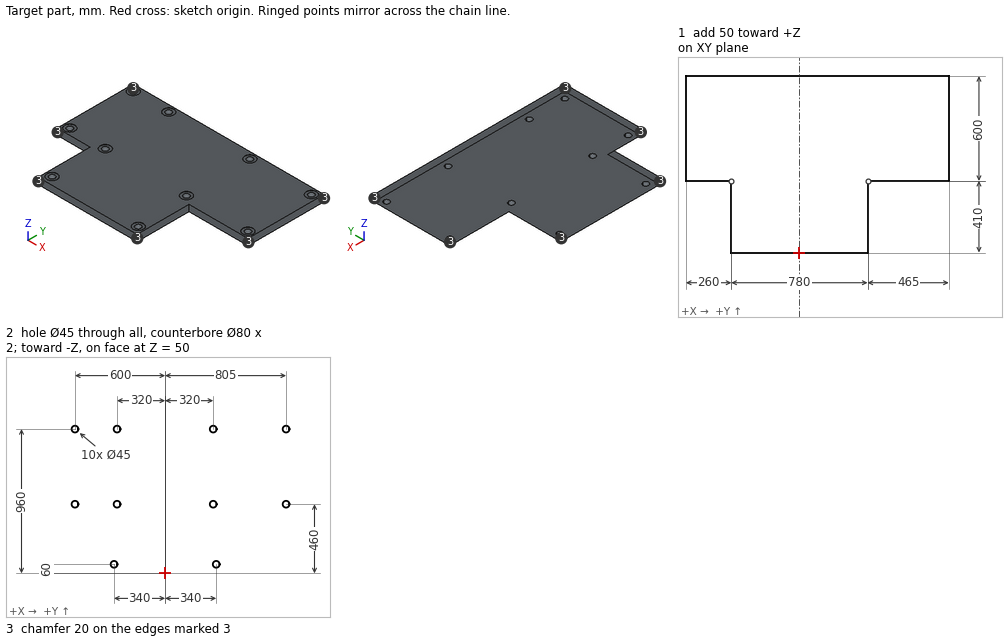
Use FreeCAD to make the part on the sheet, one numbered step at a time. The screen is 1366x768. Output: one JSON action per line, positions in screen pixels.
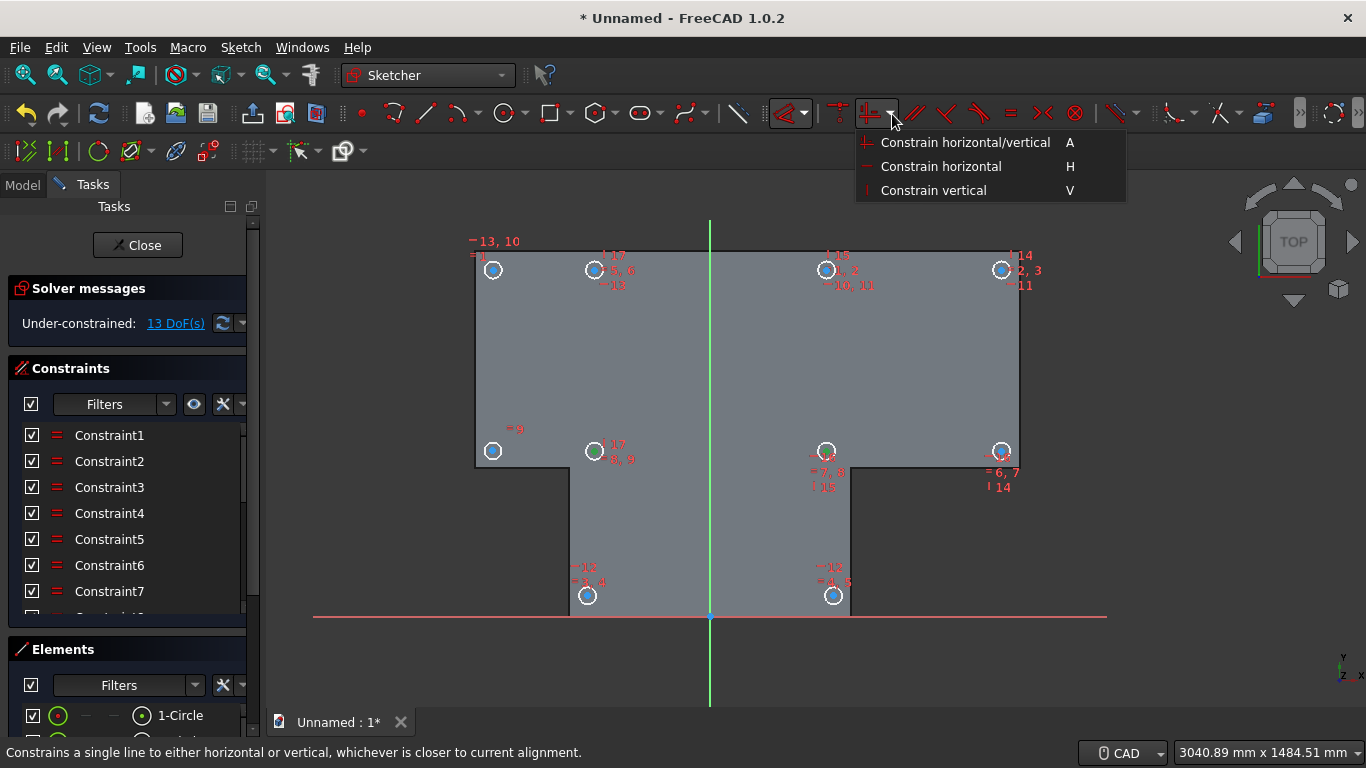
{"action": "left_click", "coordinate": [991, 166]}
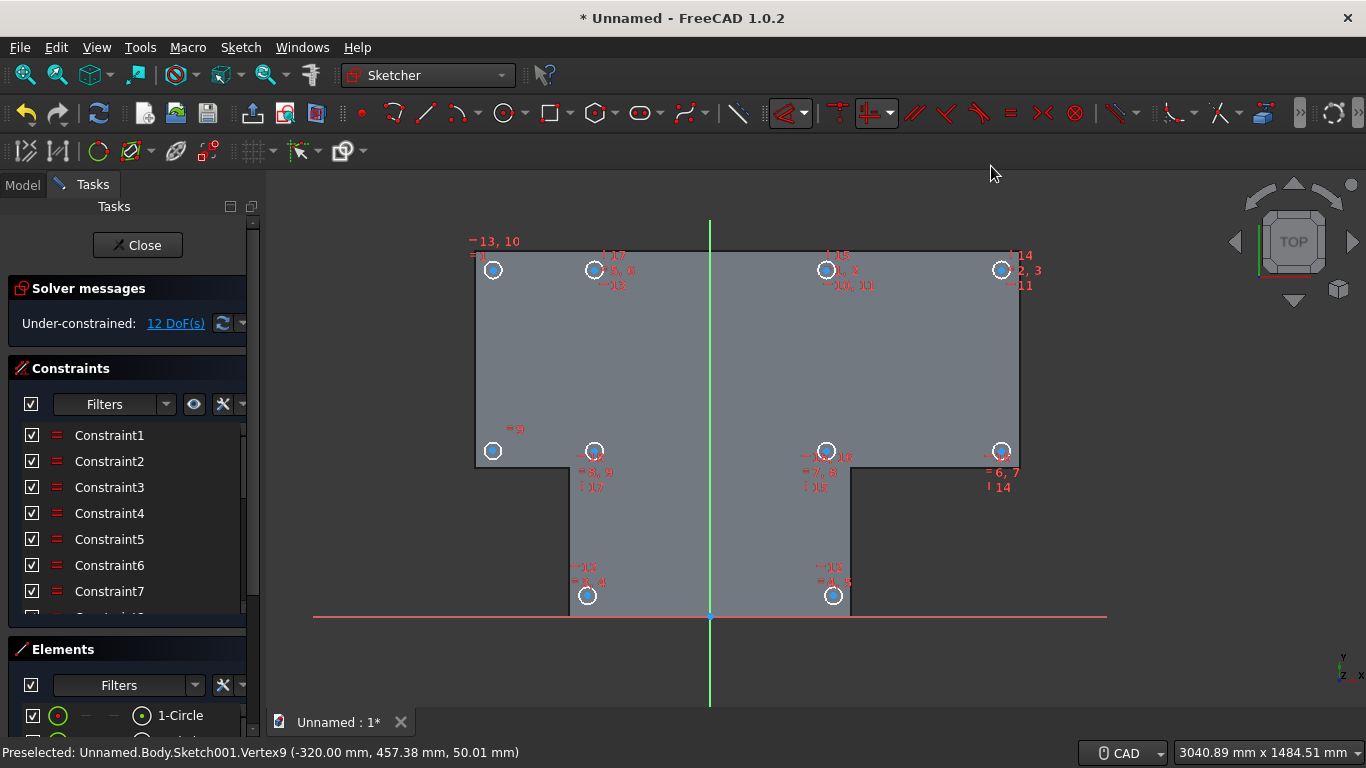
{"action": "left_click", "coordinate": [493, 270]}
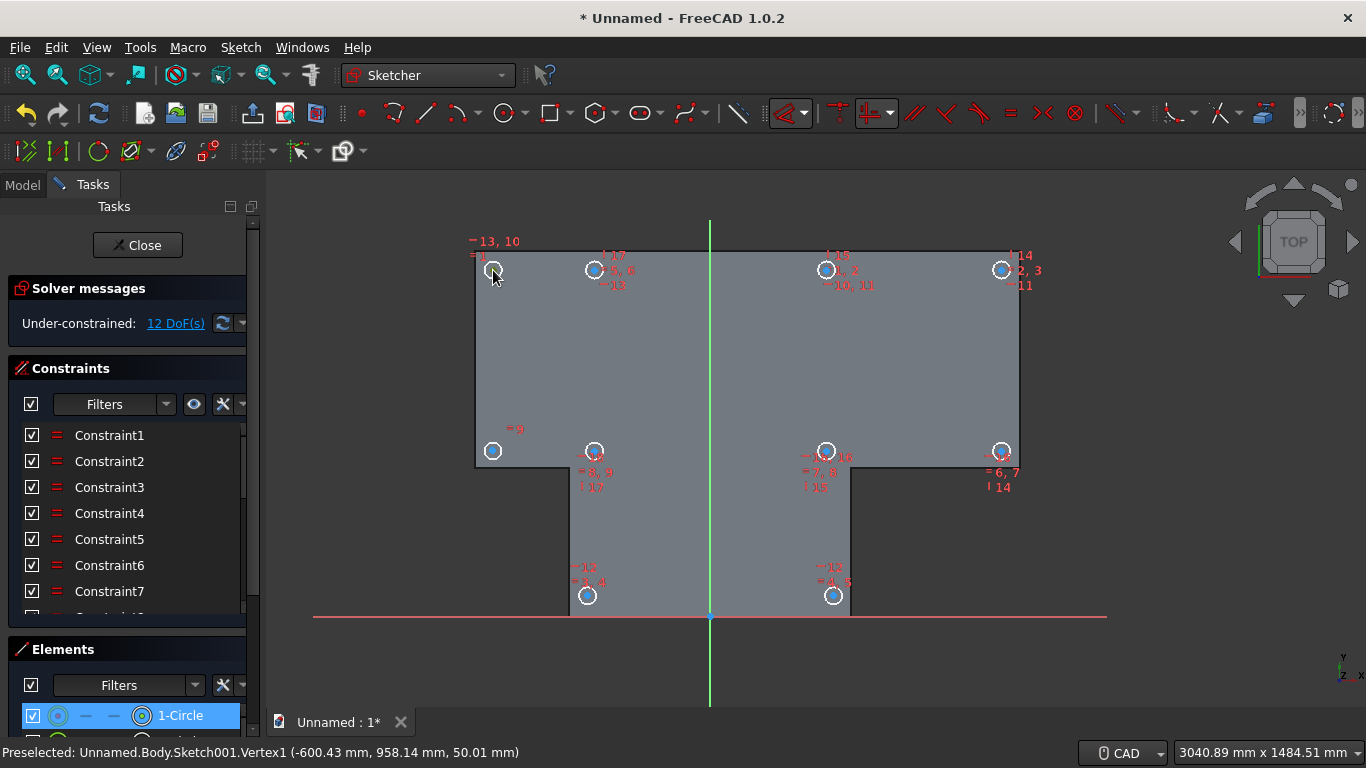
{"action": "left_click", "coordinate": [493, 451]}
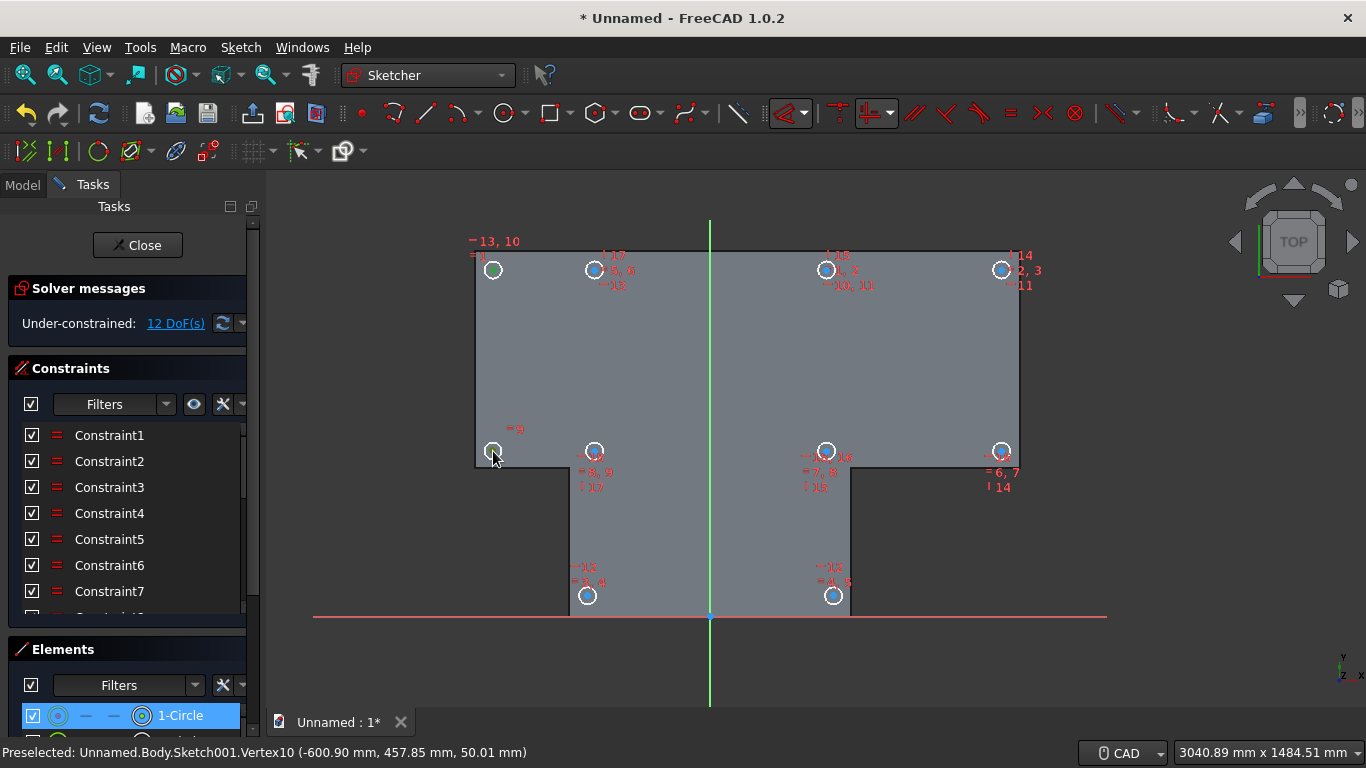
{"action": "left_click", "coordinate": [892, 114]}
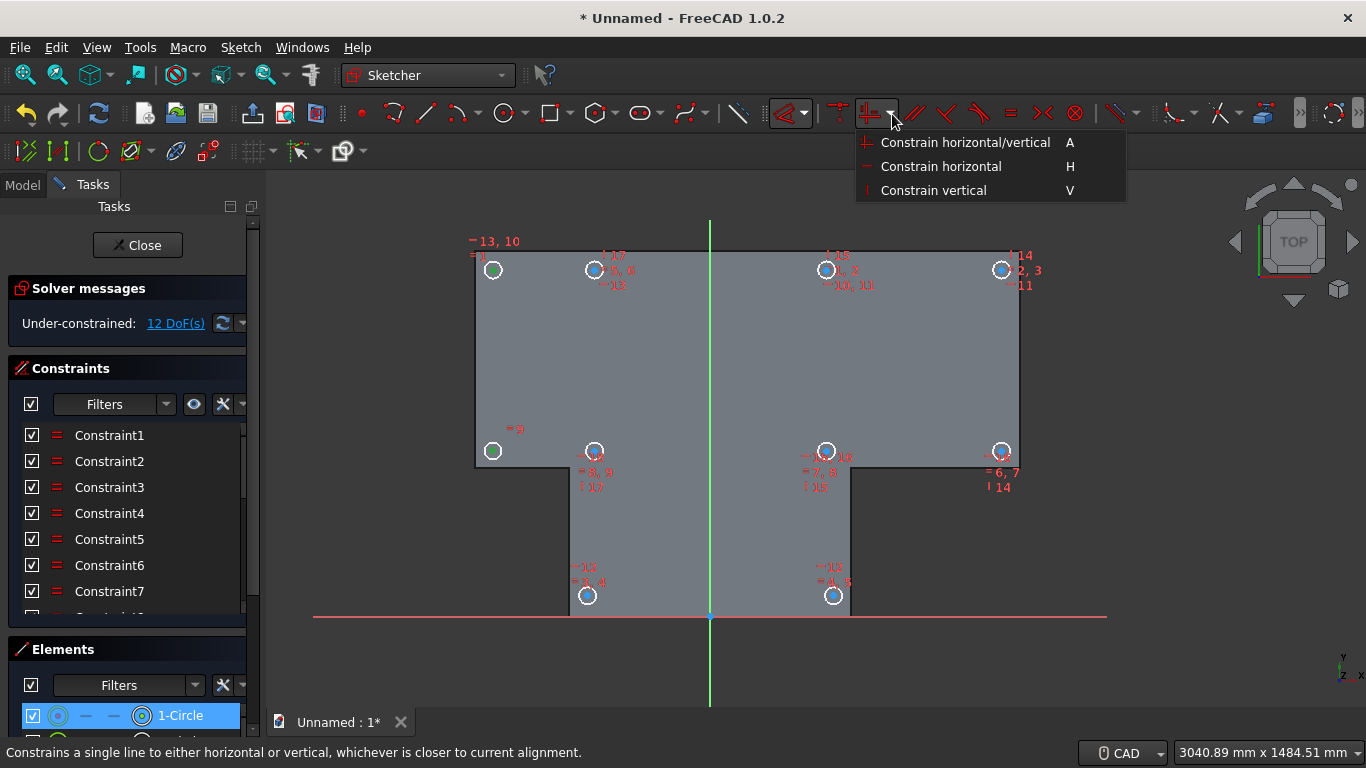
{"action": "left_click", "coordinate": [991, 190]}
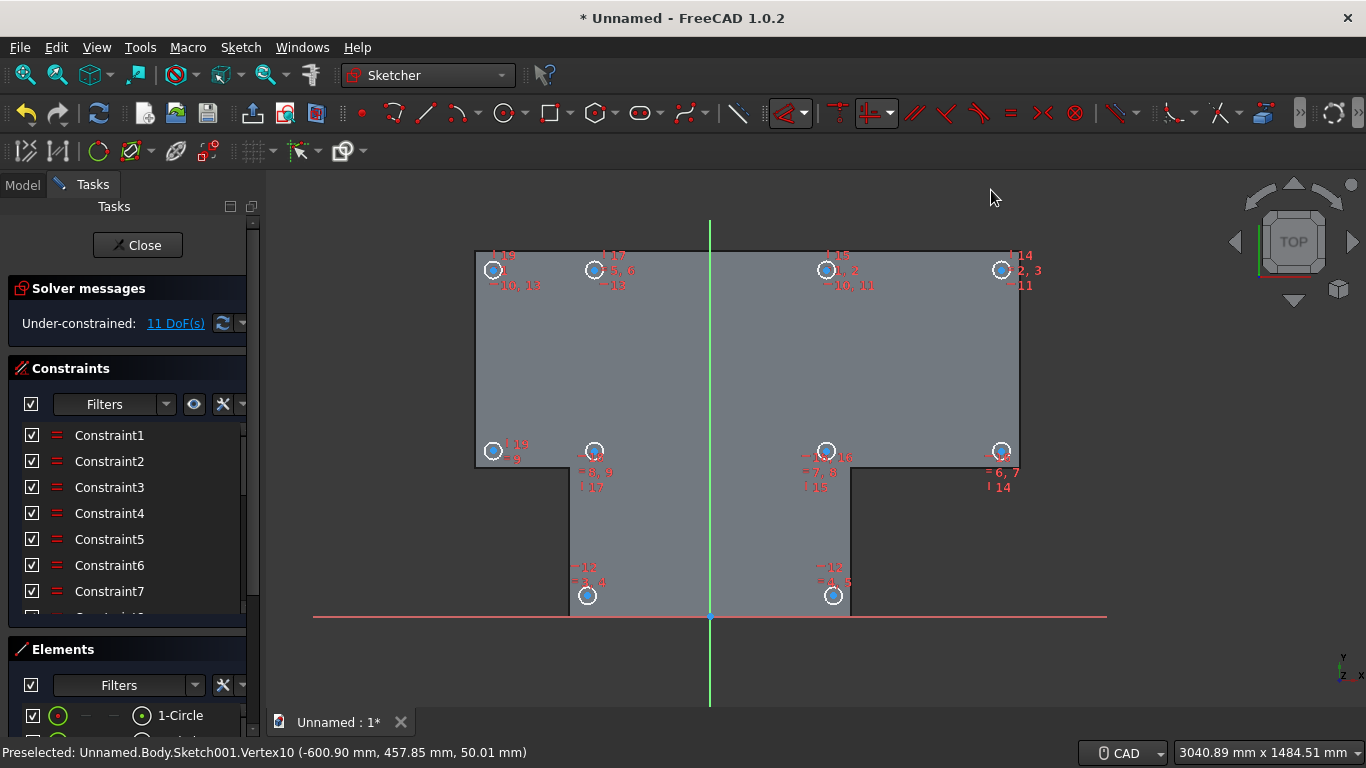
{"action": "left_click", "coordinate": [593, 449]}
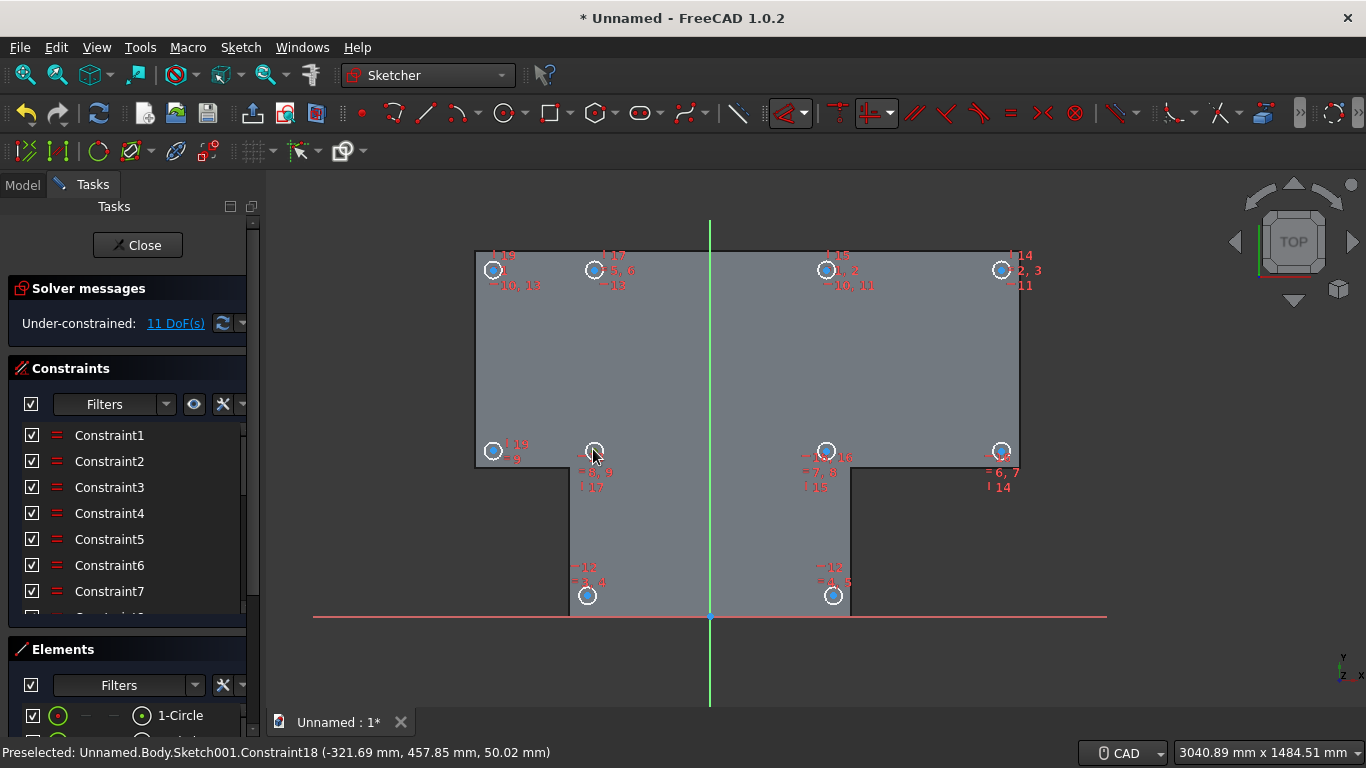
{"action": "left_click", "coordinate": [493, 451]}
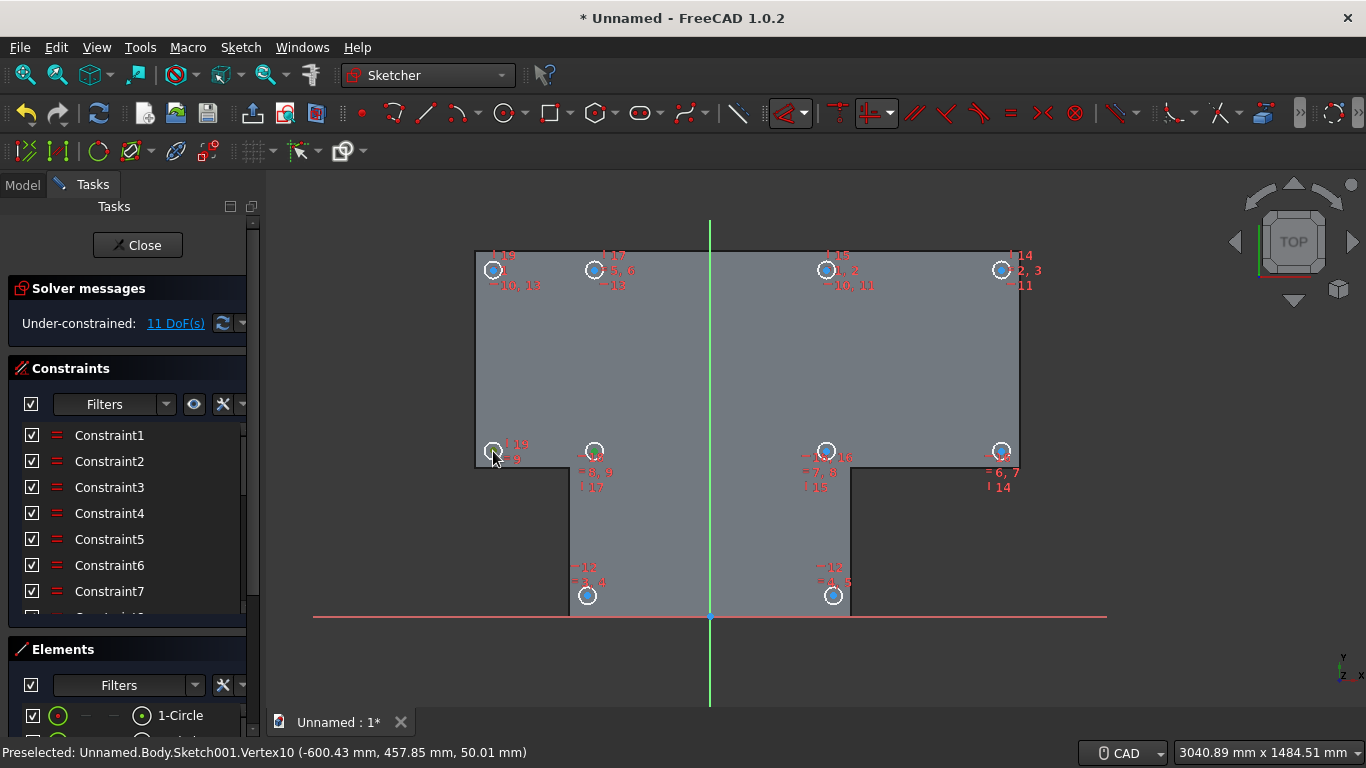
{"action": "key", "text": "h"}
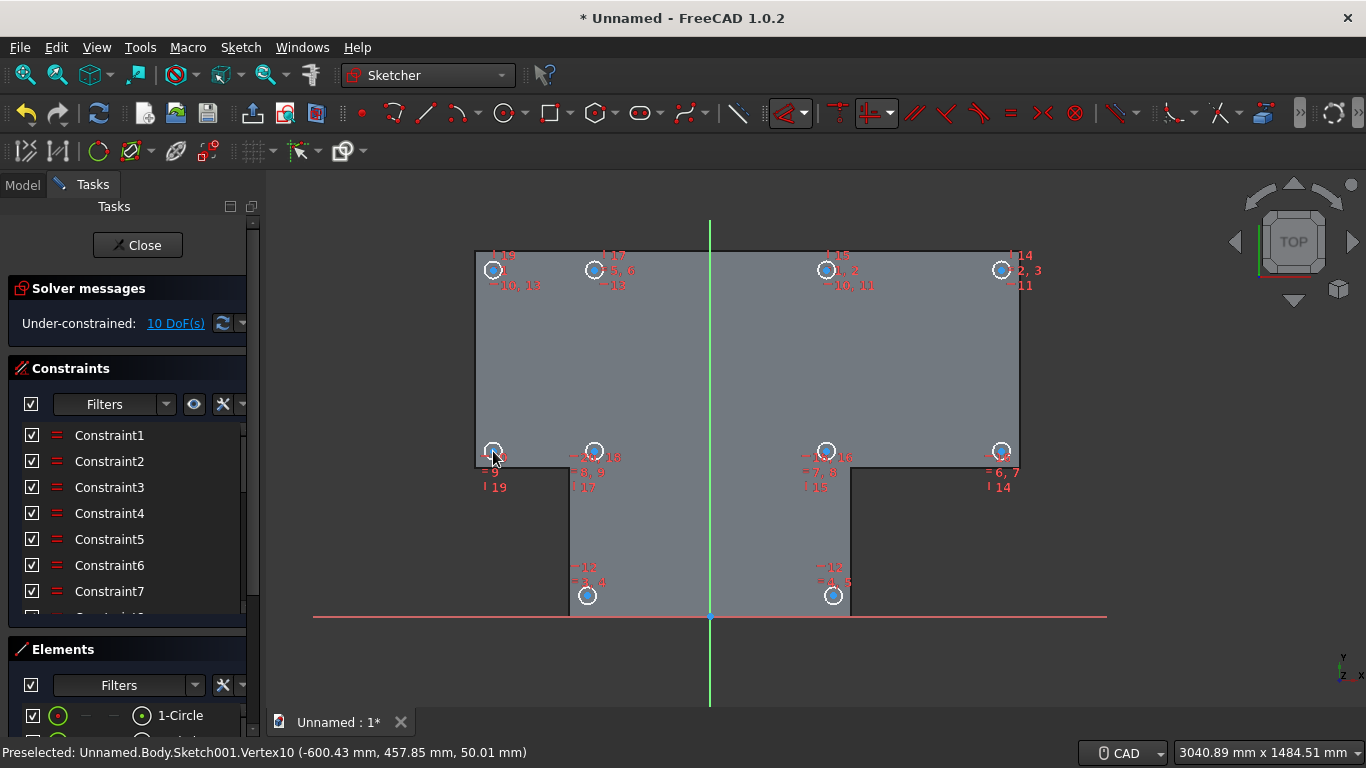
{"action": "scroll", "coordinate": [493, 262], "scroll_direction": "up", "scroll_amount": 5}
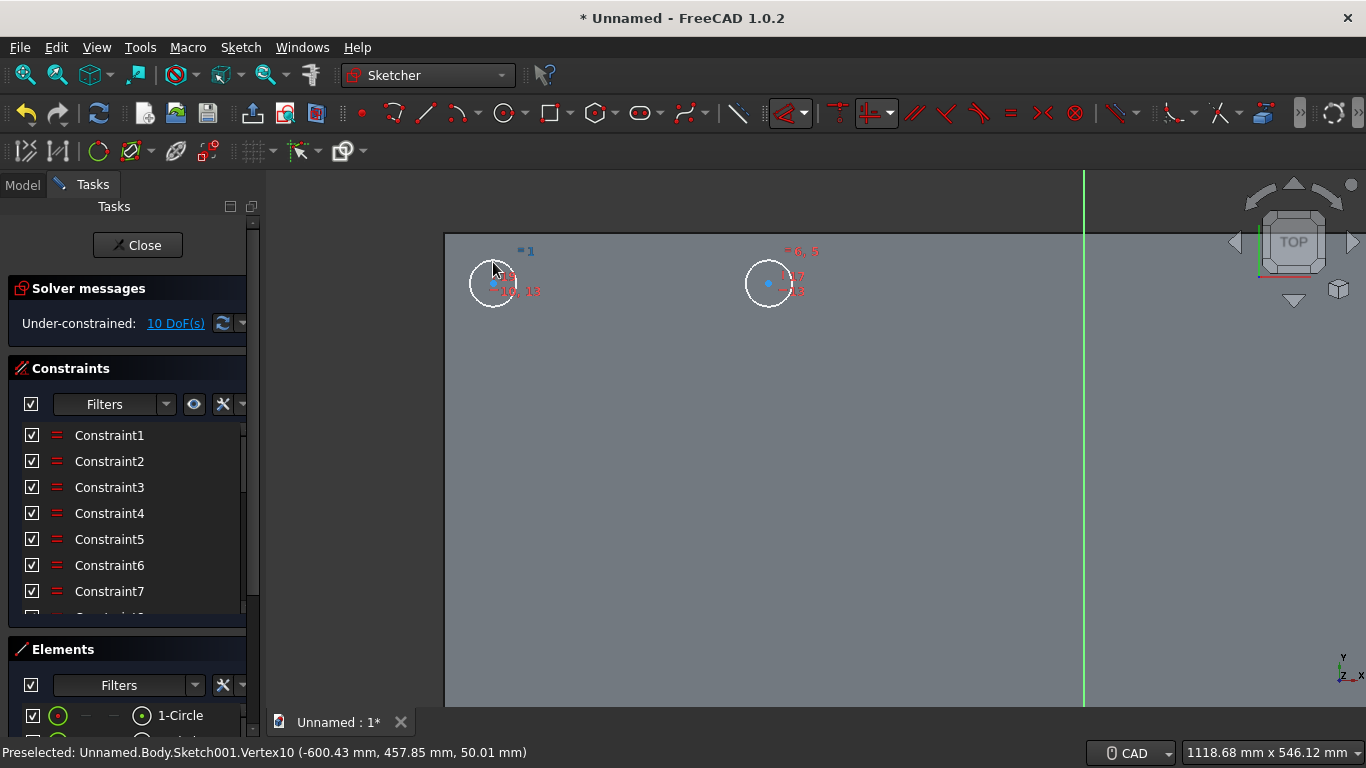
{"action": "left_click", "coordinate": [494, 260]}